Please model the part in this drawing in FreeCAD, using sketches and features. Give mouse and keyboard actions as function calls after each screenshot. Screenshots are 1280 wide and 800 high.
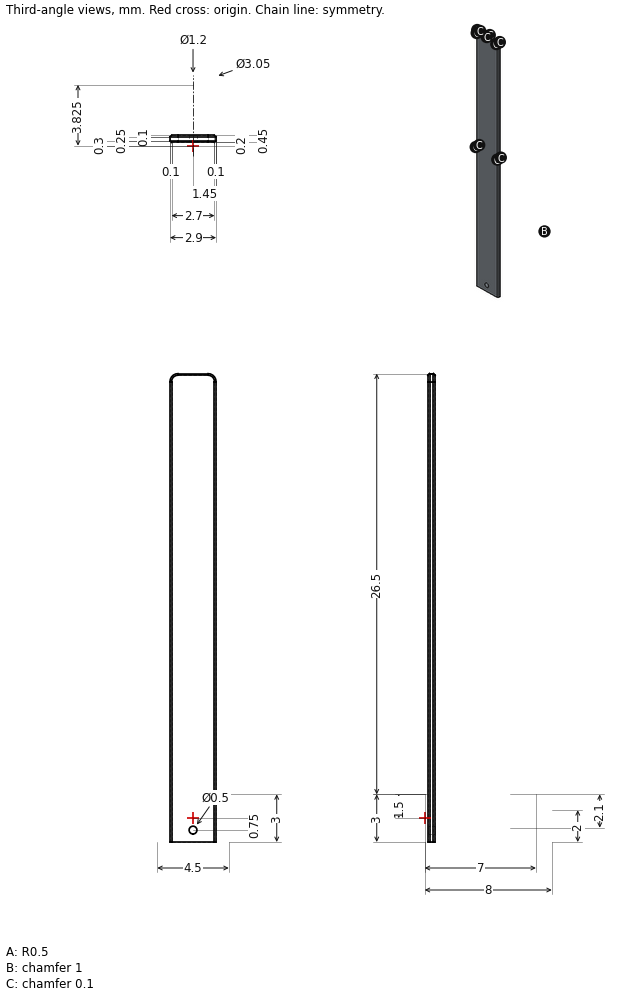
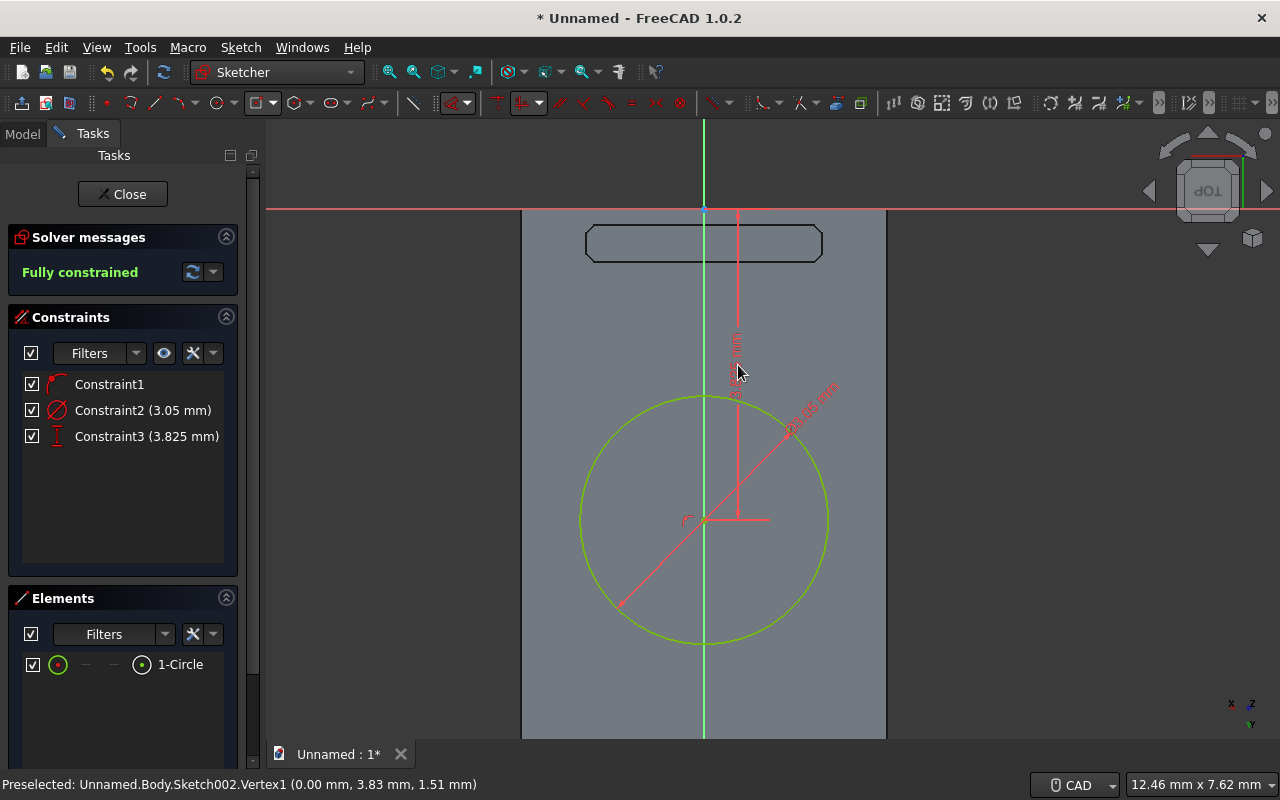
click(123, 194)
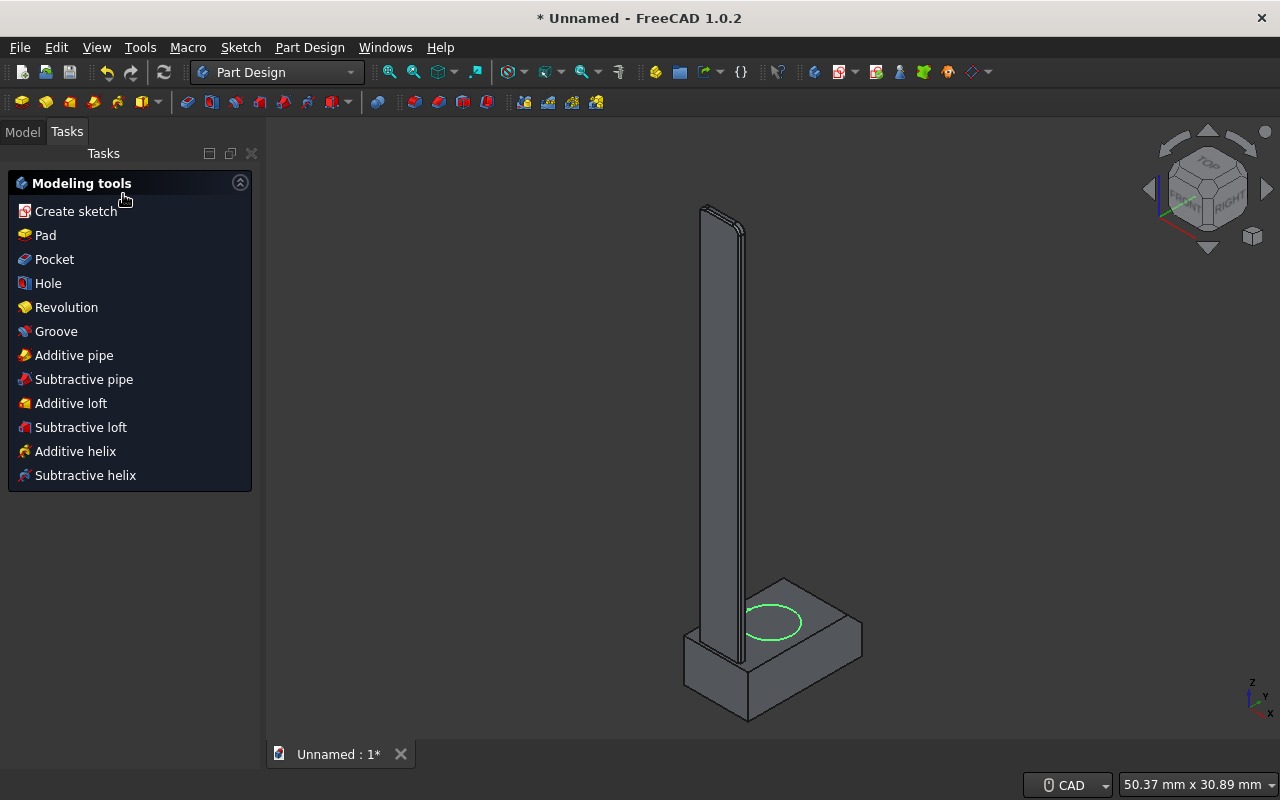
click(188, 102)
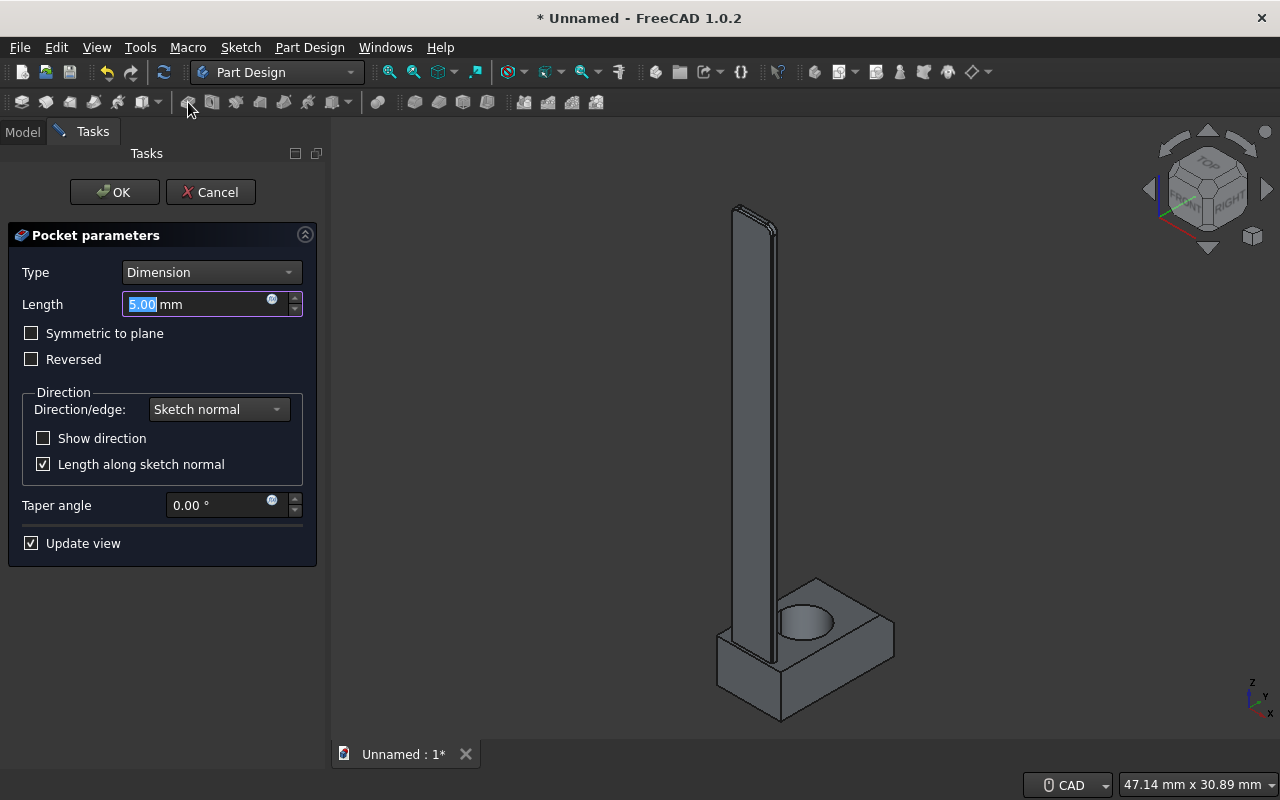
text(2.1)
key(Tab)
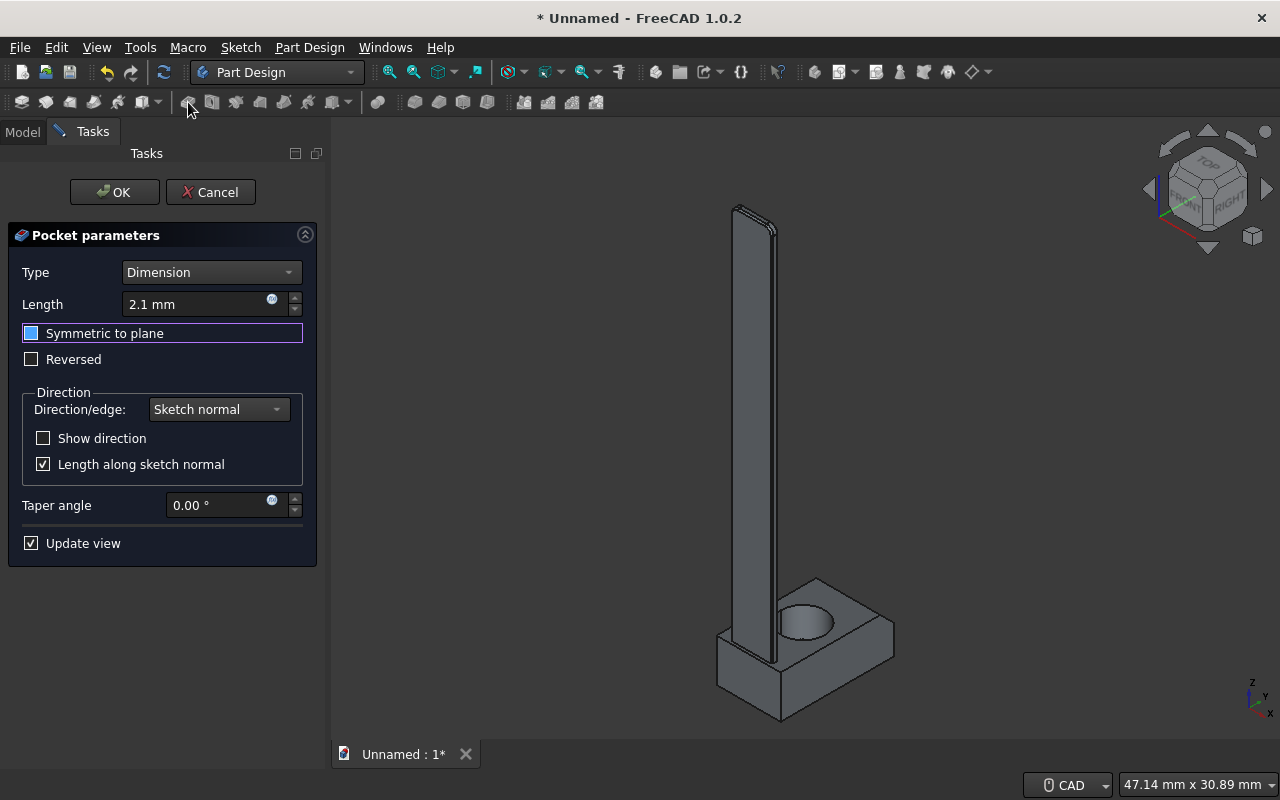
click(115, 192)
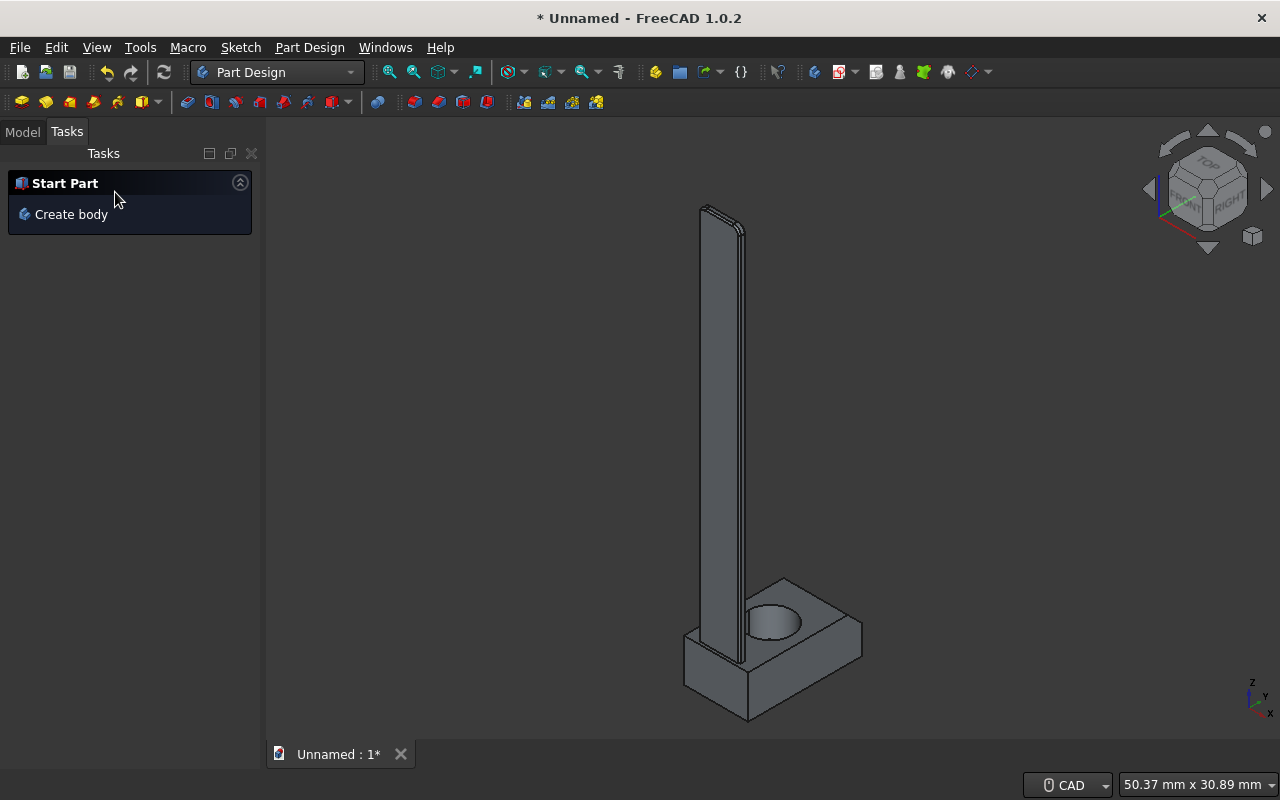
key(2)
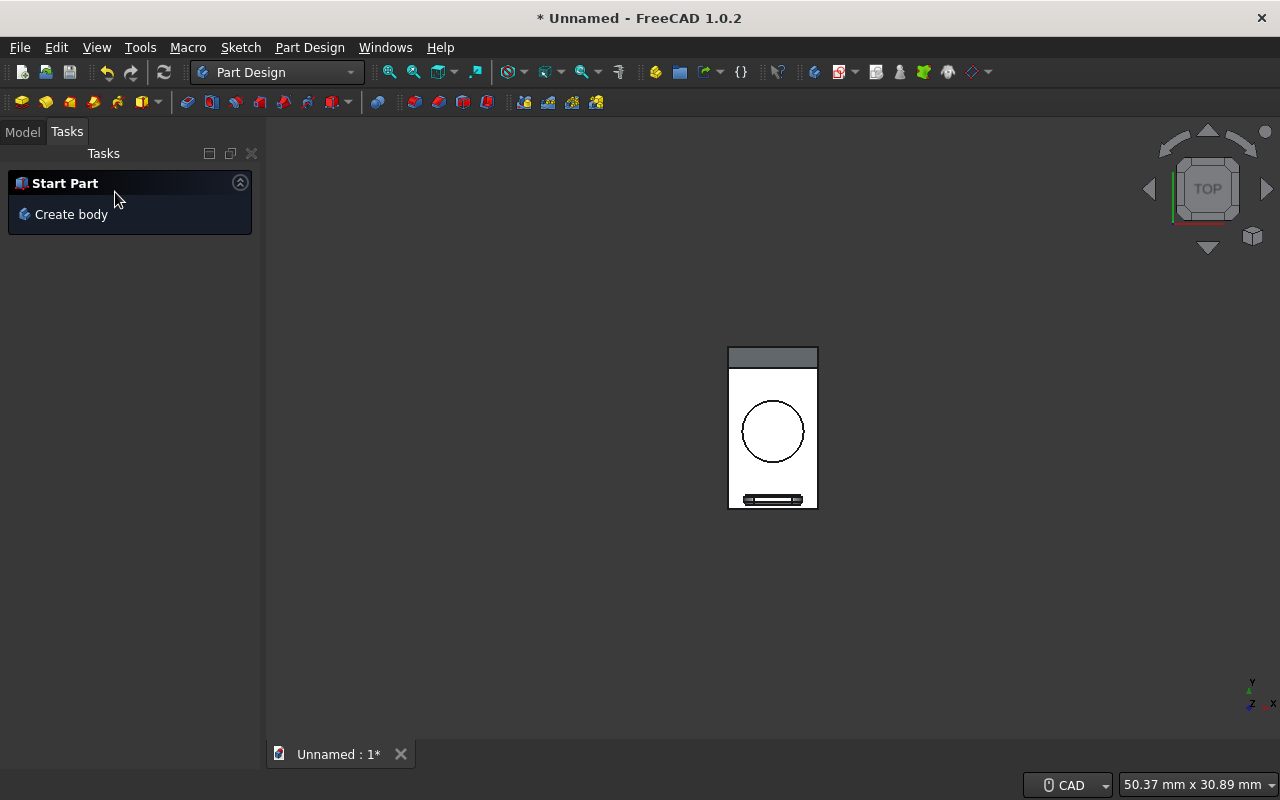
key(v)
key(f)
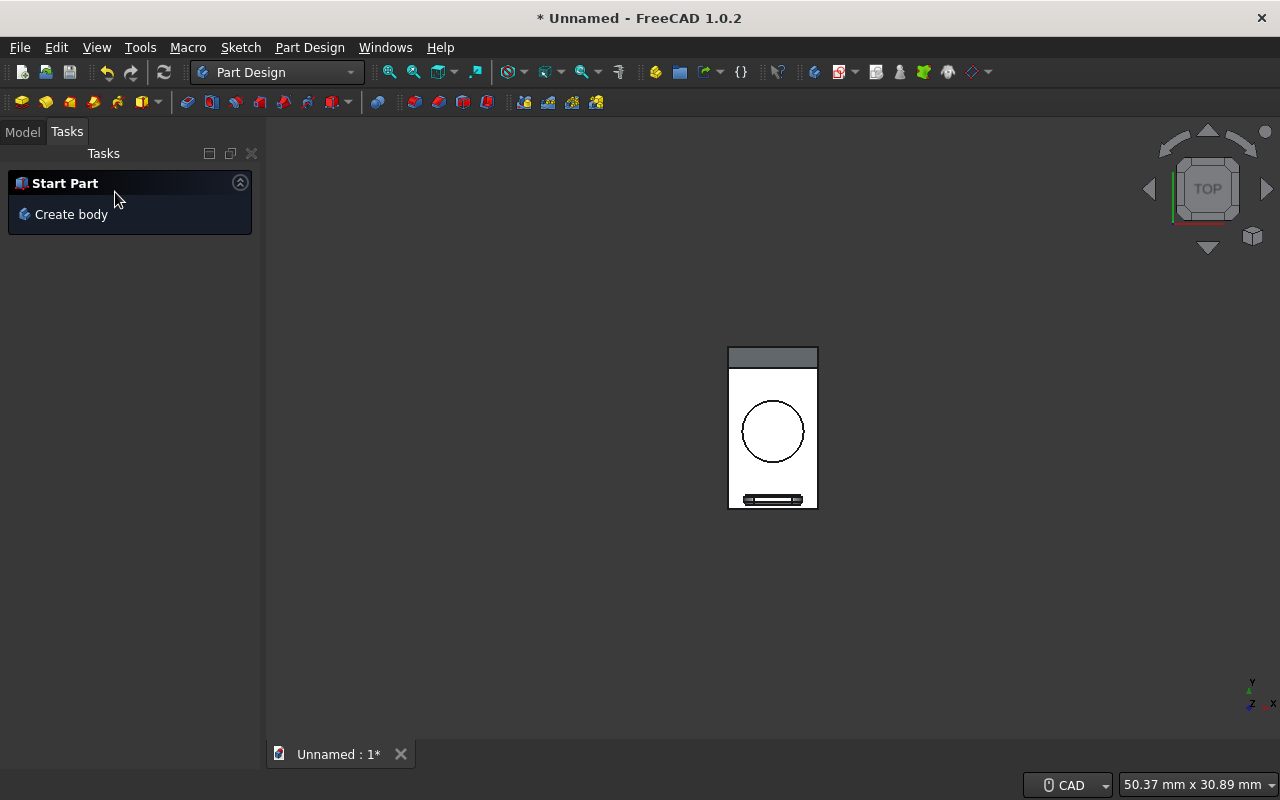
click(773, 431)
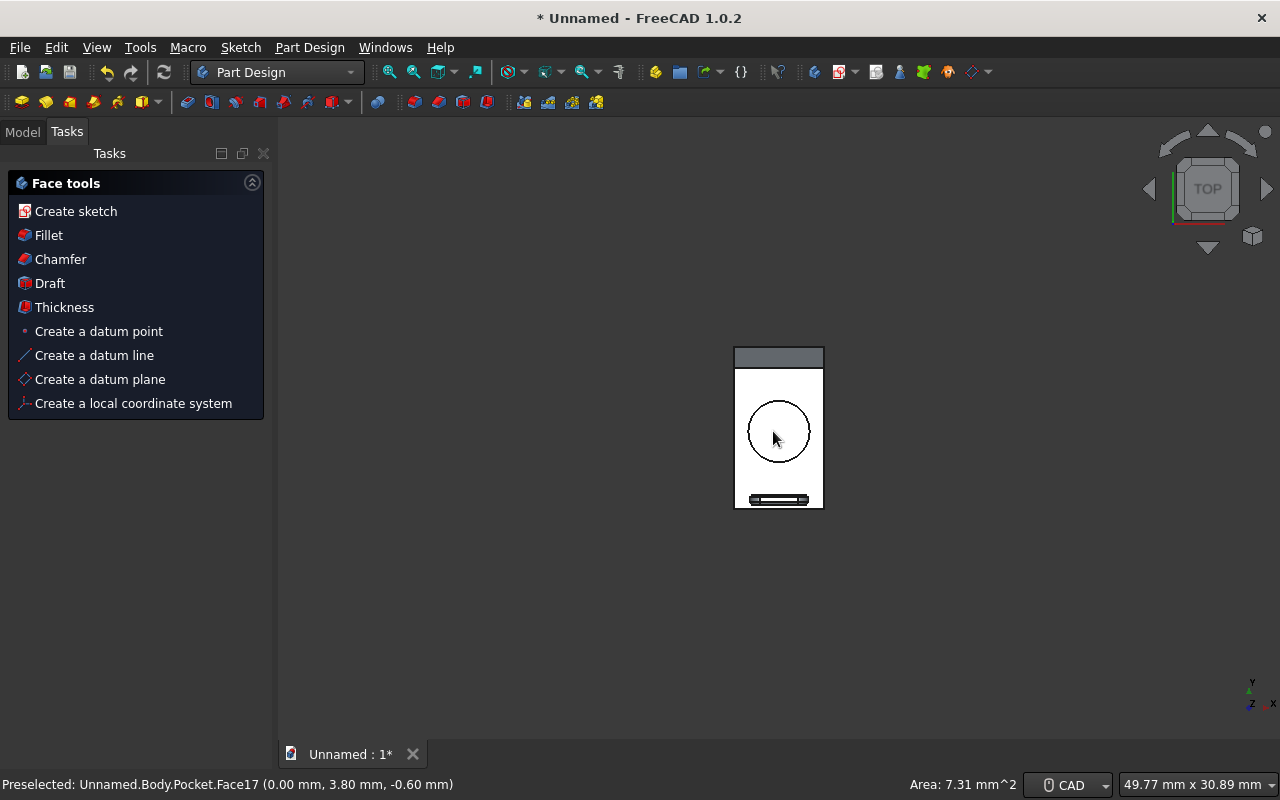
click(840, 72)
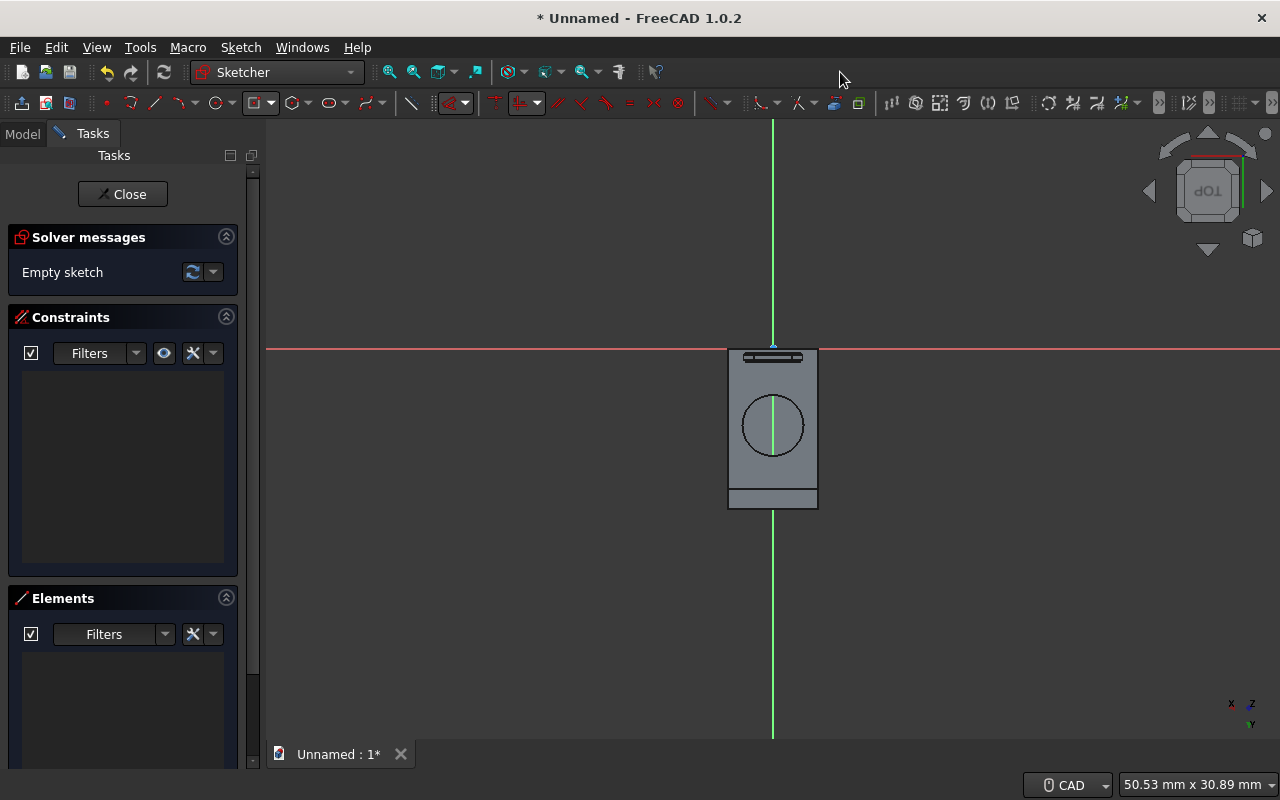
scroll(777, 425, up, 14)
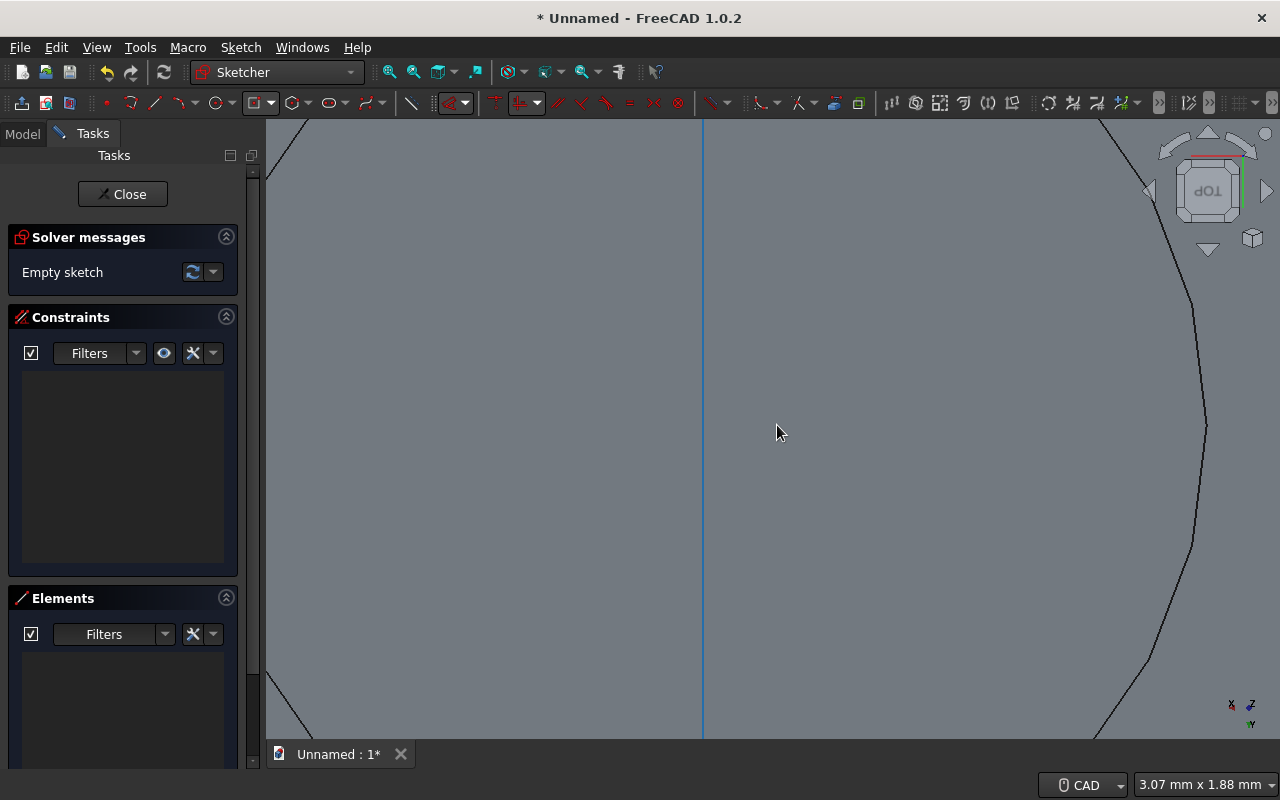
click(216, 104)